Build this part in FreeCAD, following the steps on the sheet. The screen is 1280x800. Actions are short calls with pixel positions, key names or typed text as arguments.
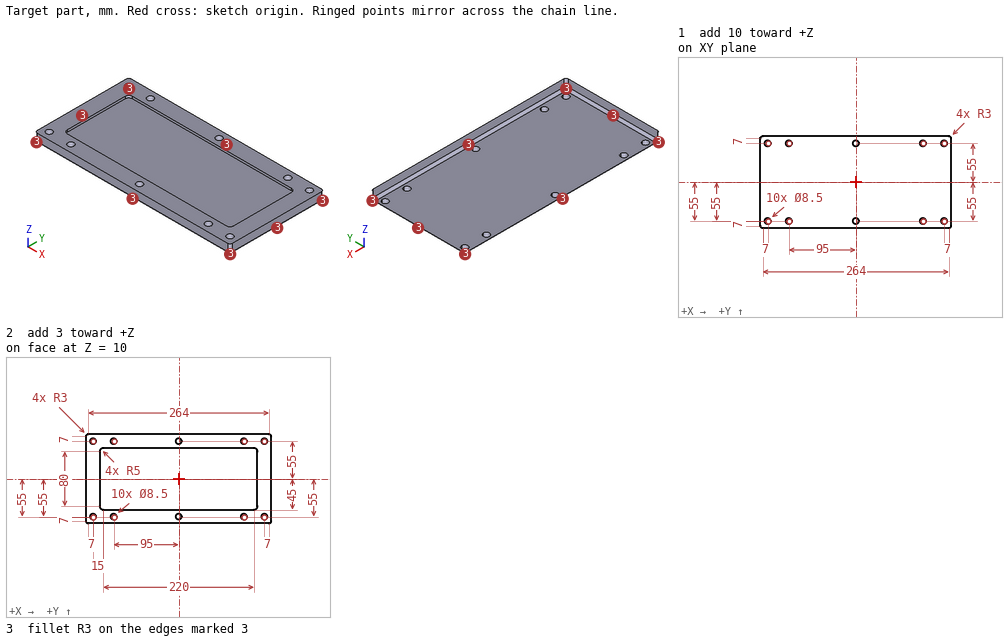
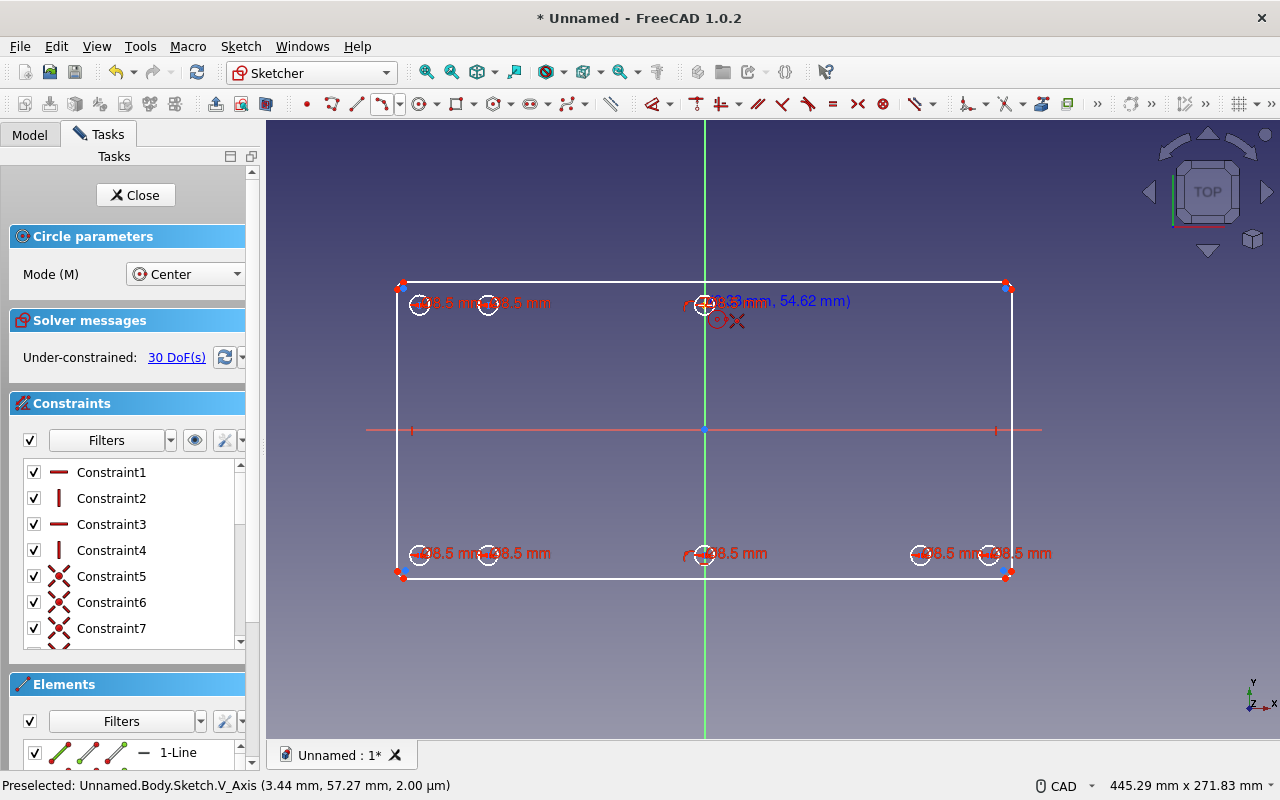
scroll(921, 305, up, 5)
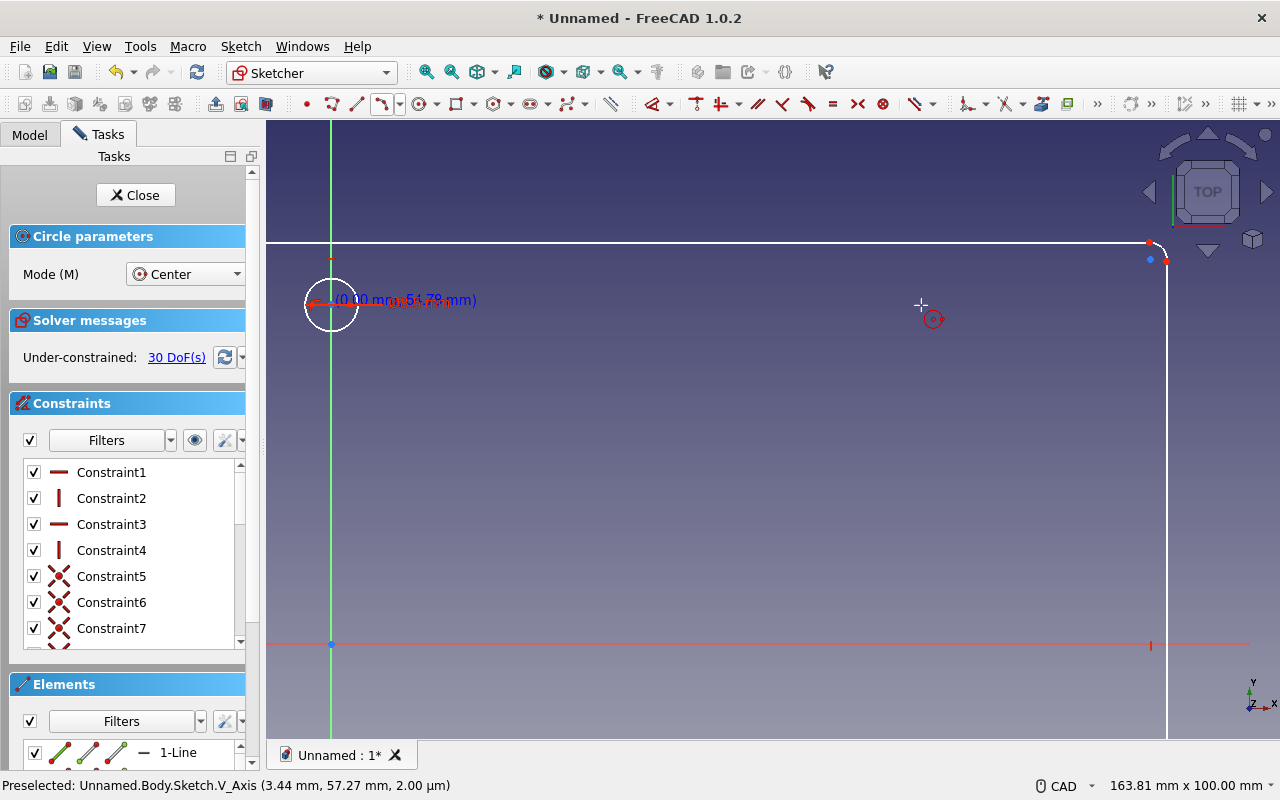
click(919, 304)
move(938, 285)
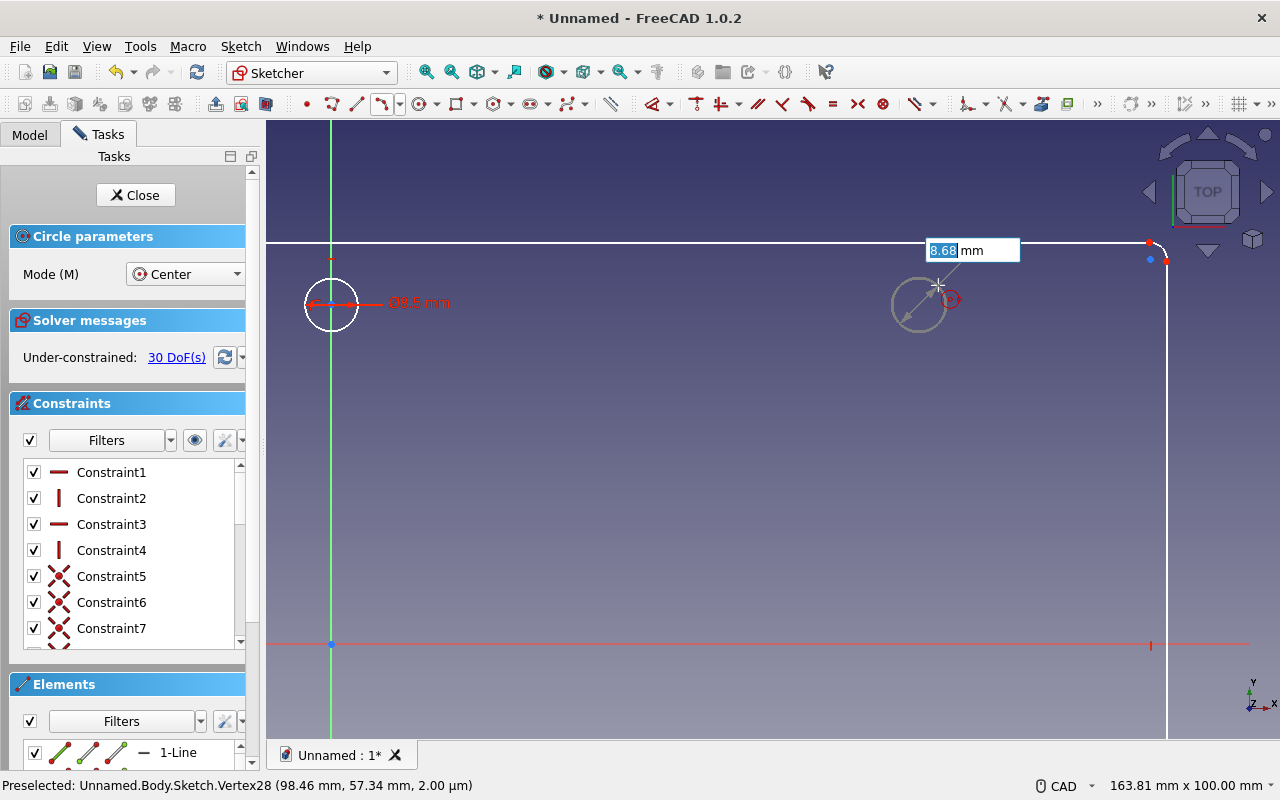
text(8.5)
key(Return)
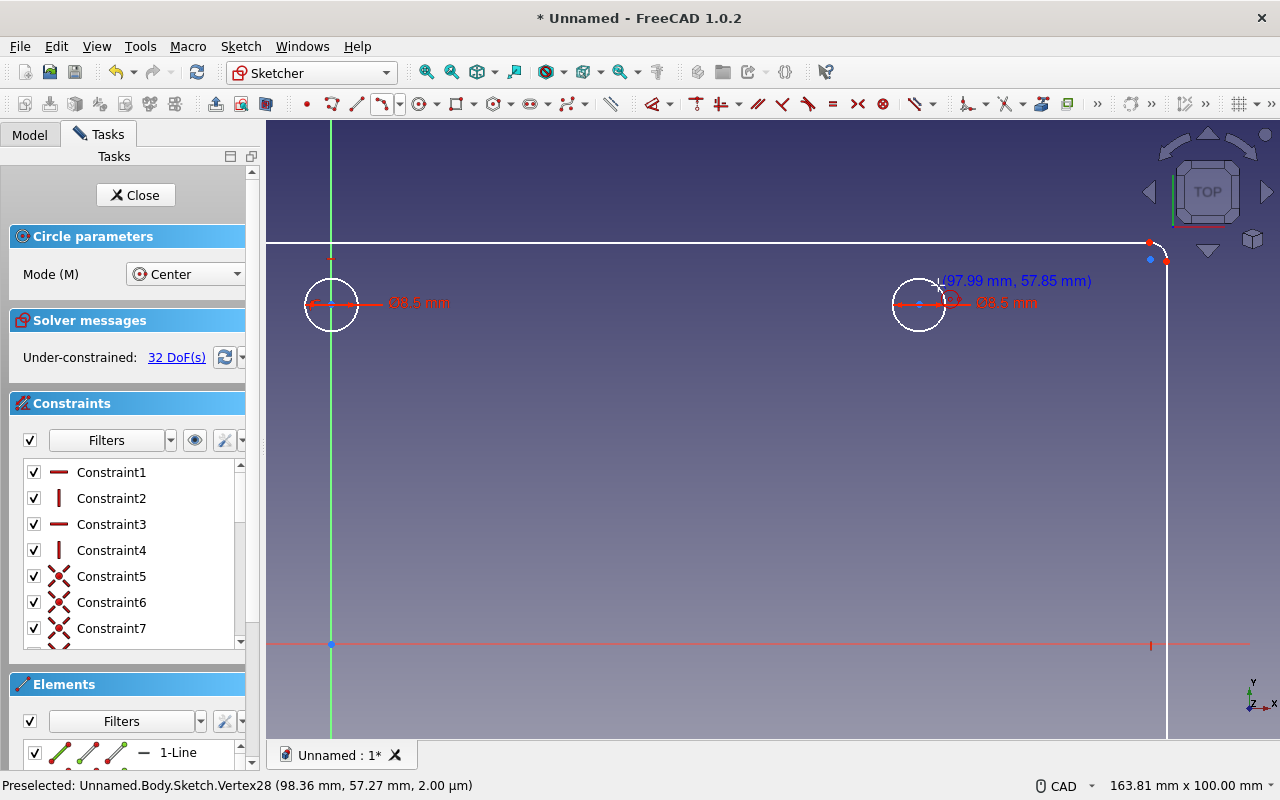
click(1105, 304)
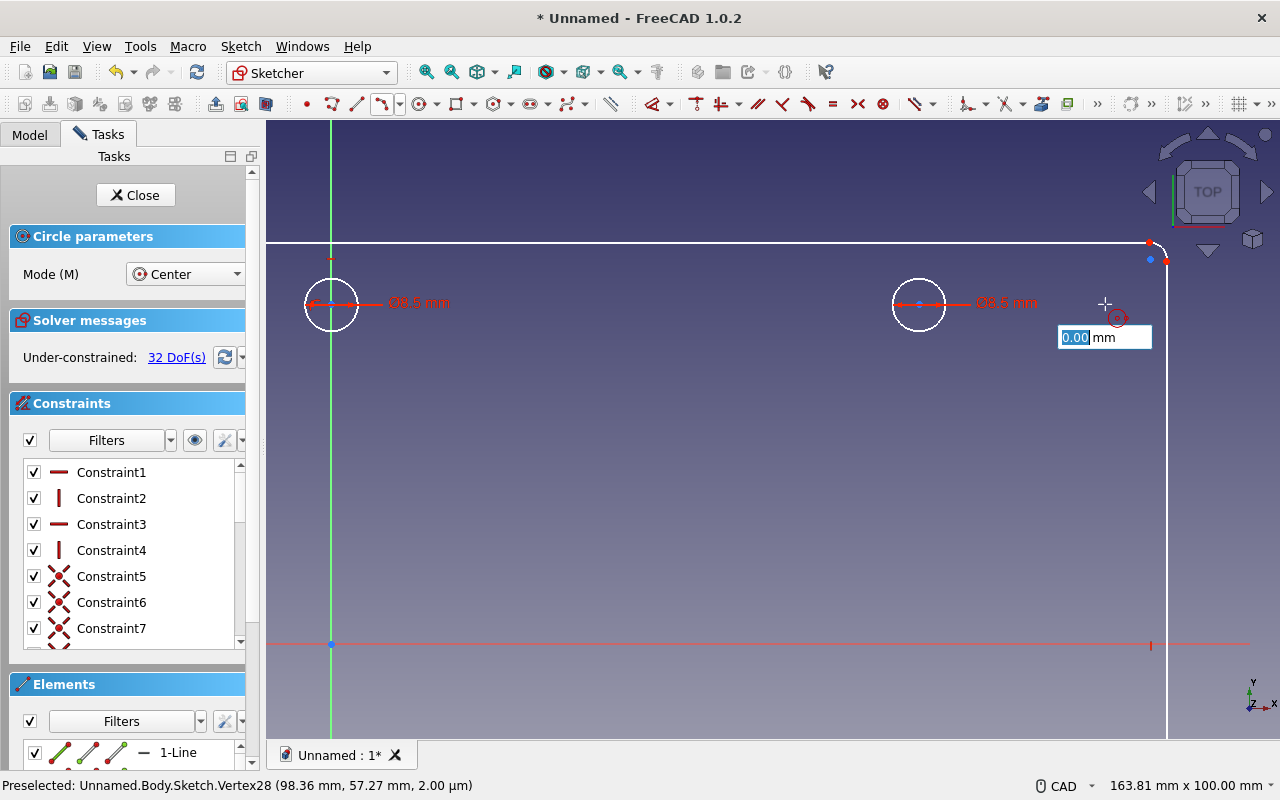
scroll(922, 305, down, 5)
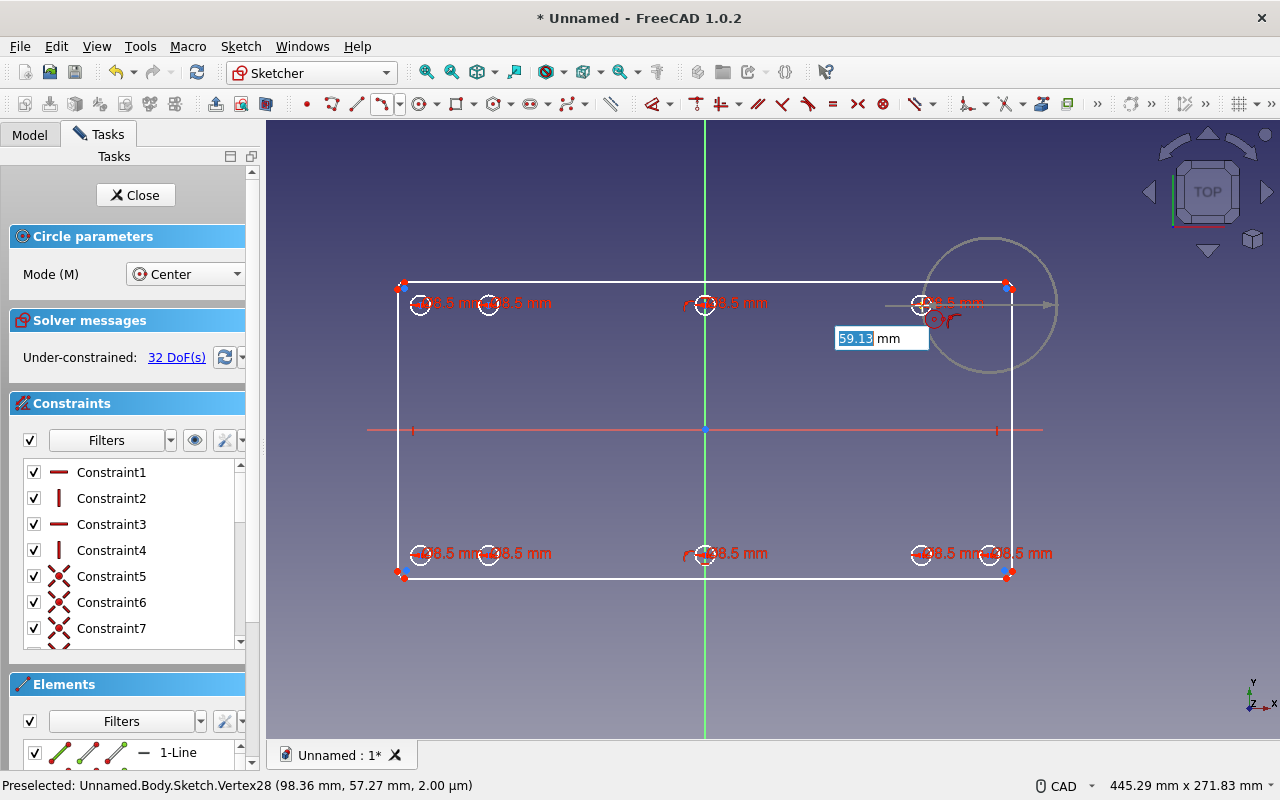
scroll(997, 298, up, 2)
move(996, 298)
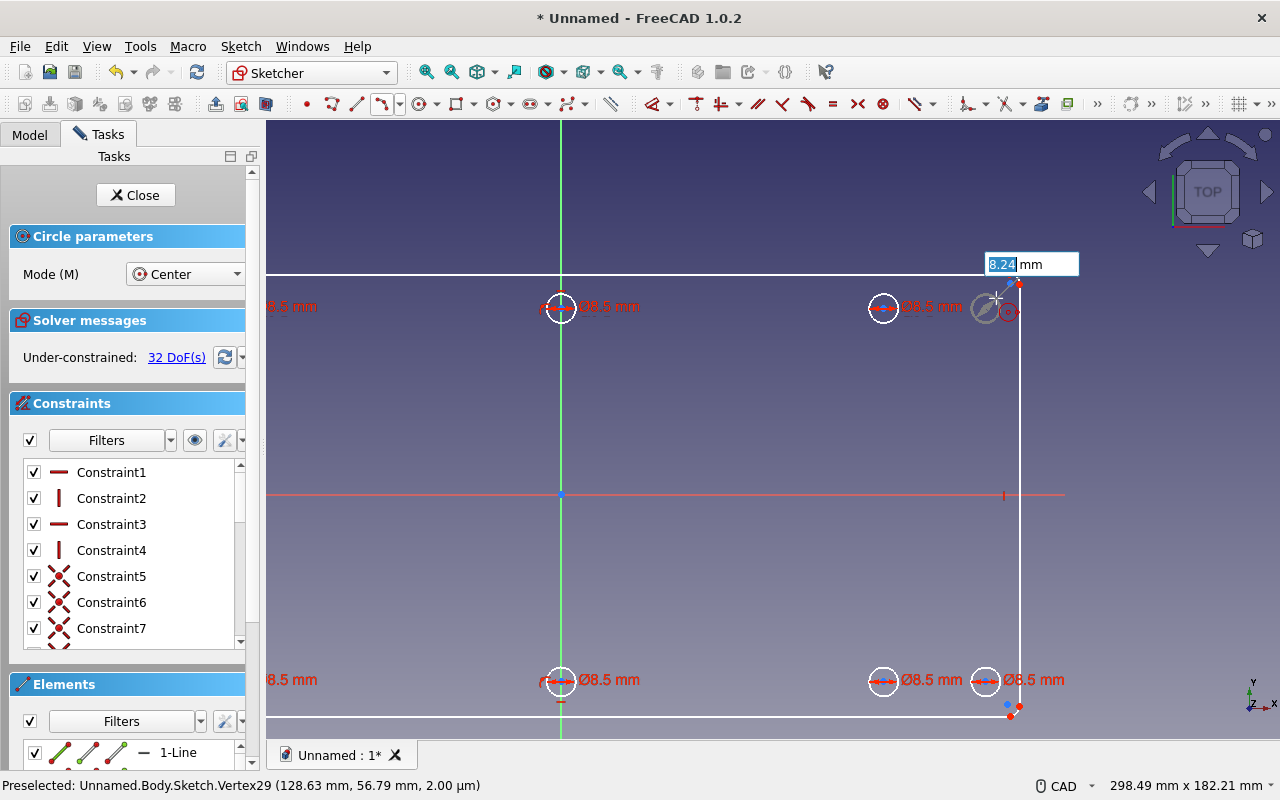
text(8.5)
key(Return)
key(Escape)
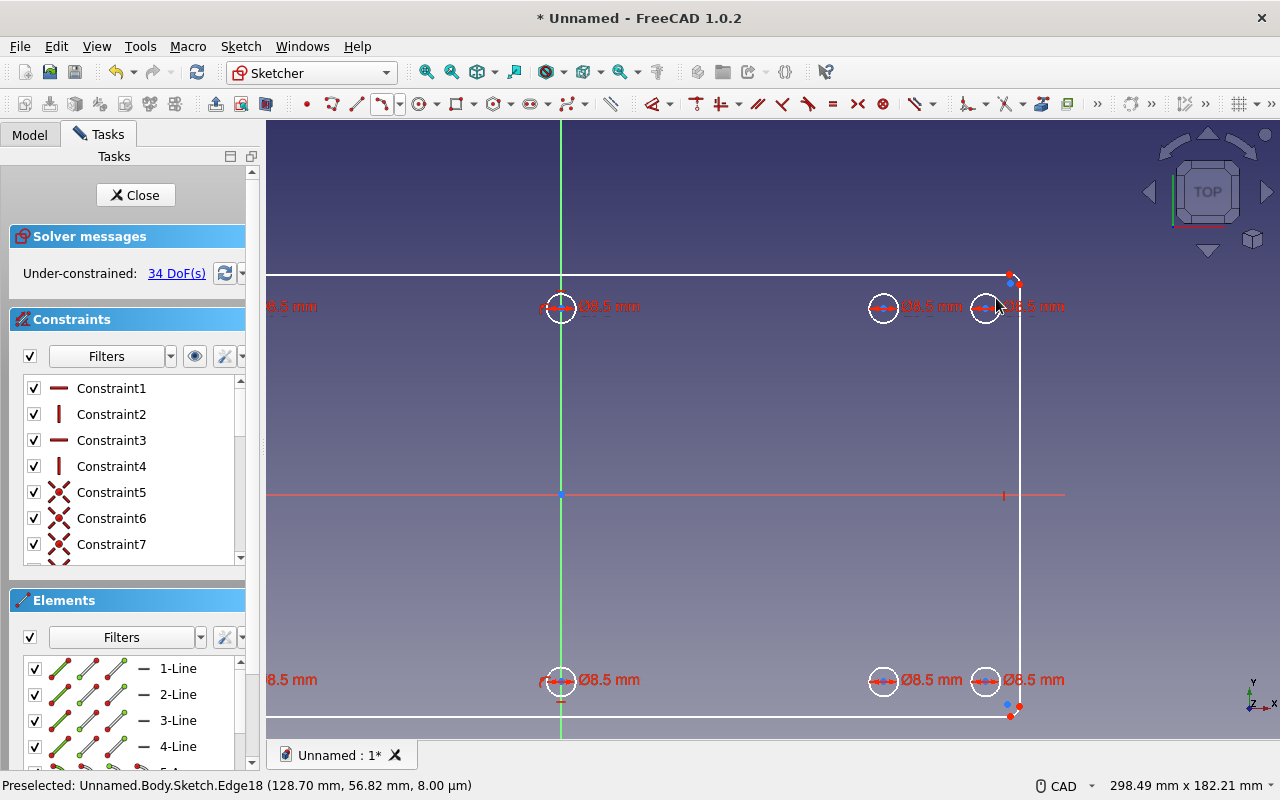
scroll(996, 297, down, 2)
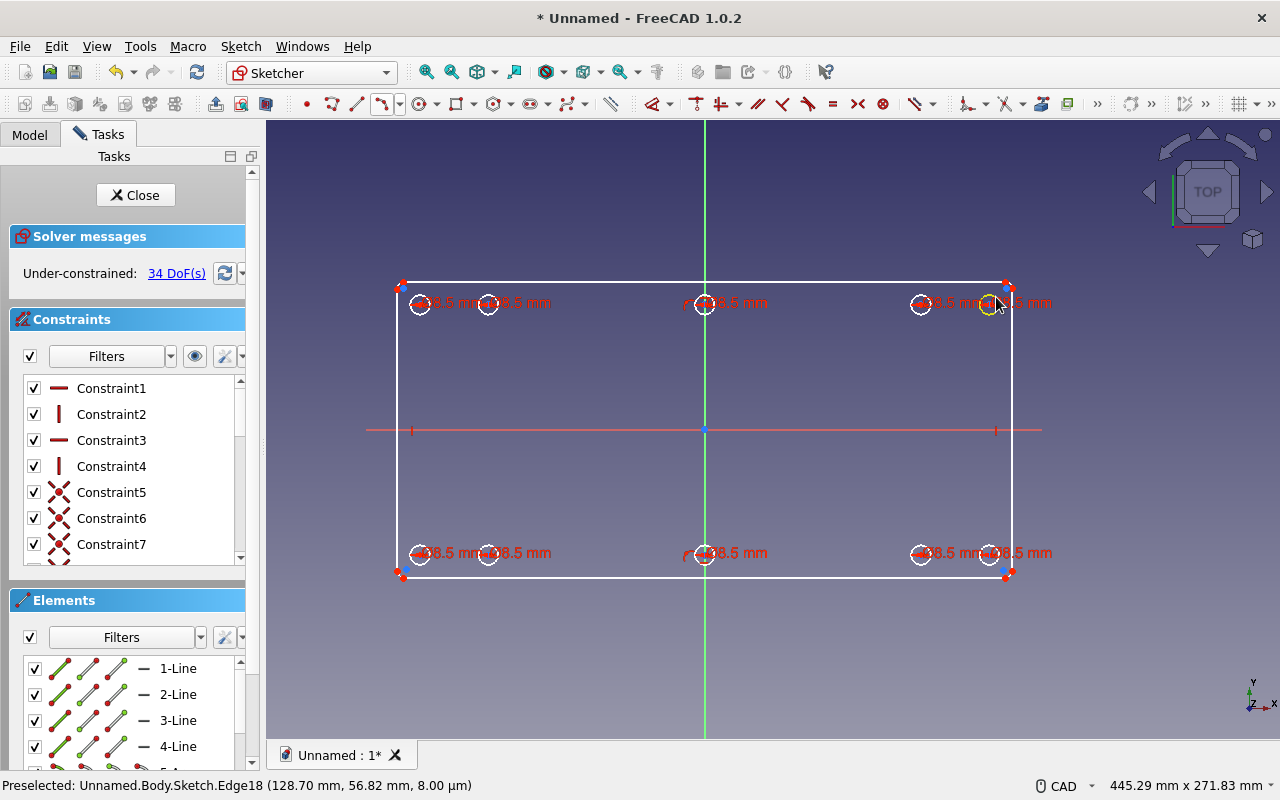
click(584, 578)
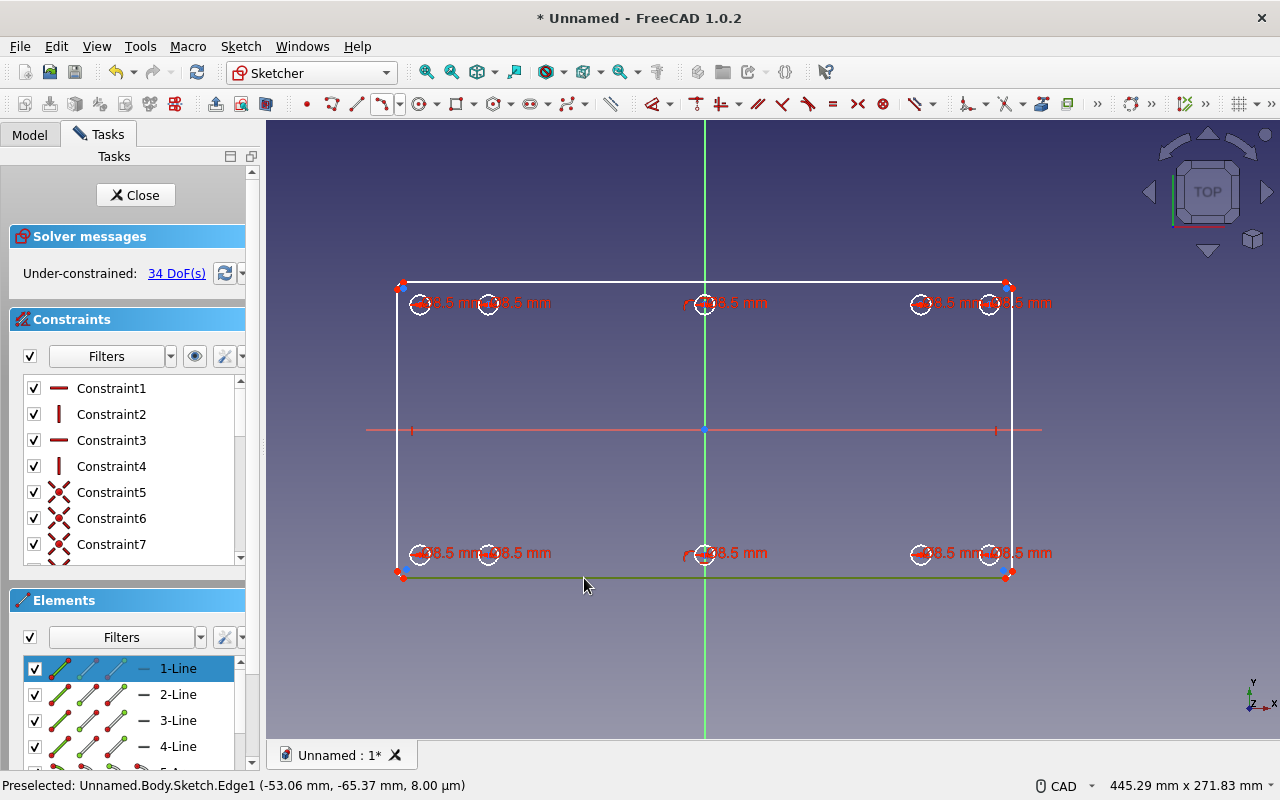
scroll(1010, 576, up, 6)